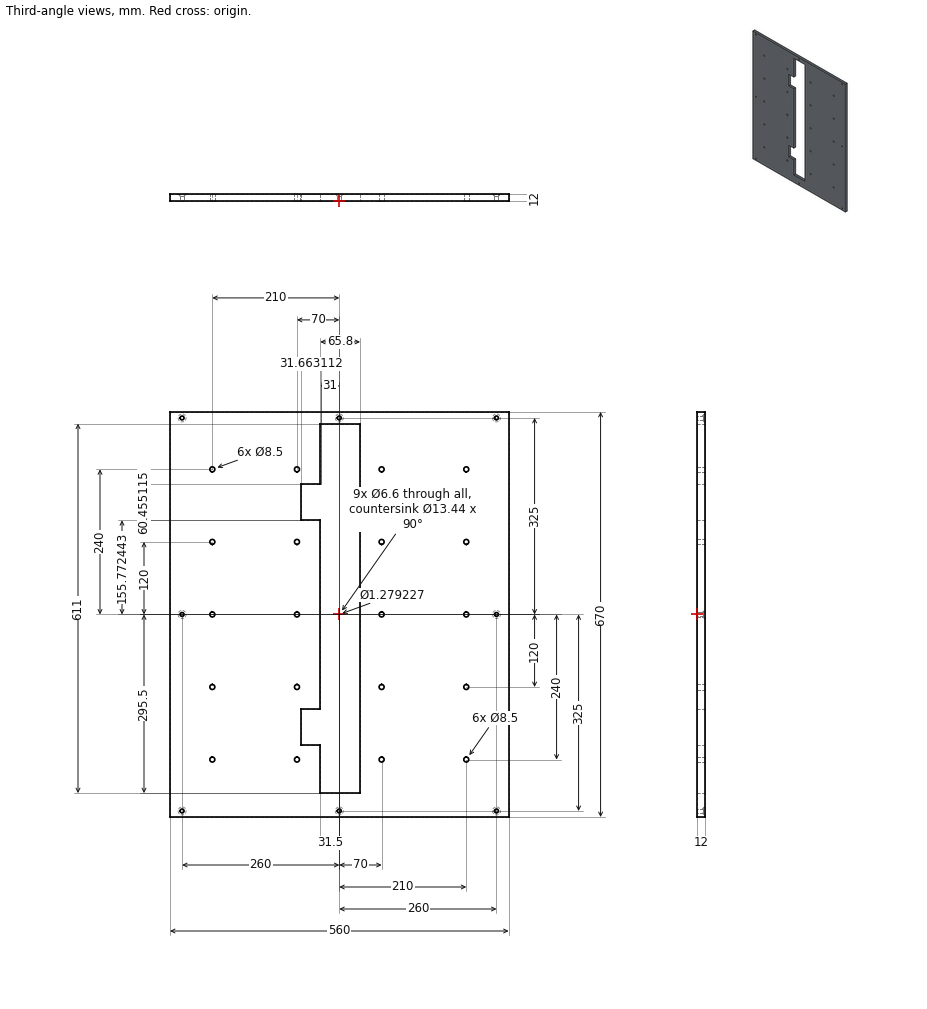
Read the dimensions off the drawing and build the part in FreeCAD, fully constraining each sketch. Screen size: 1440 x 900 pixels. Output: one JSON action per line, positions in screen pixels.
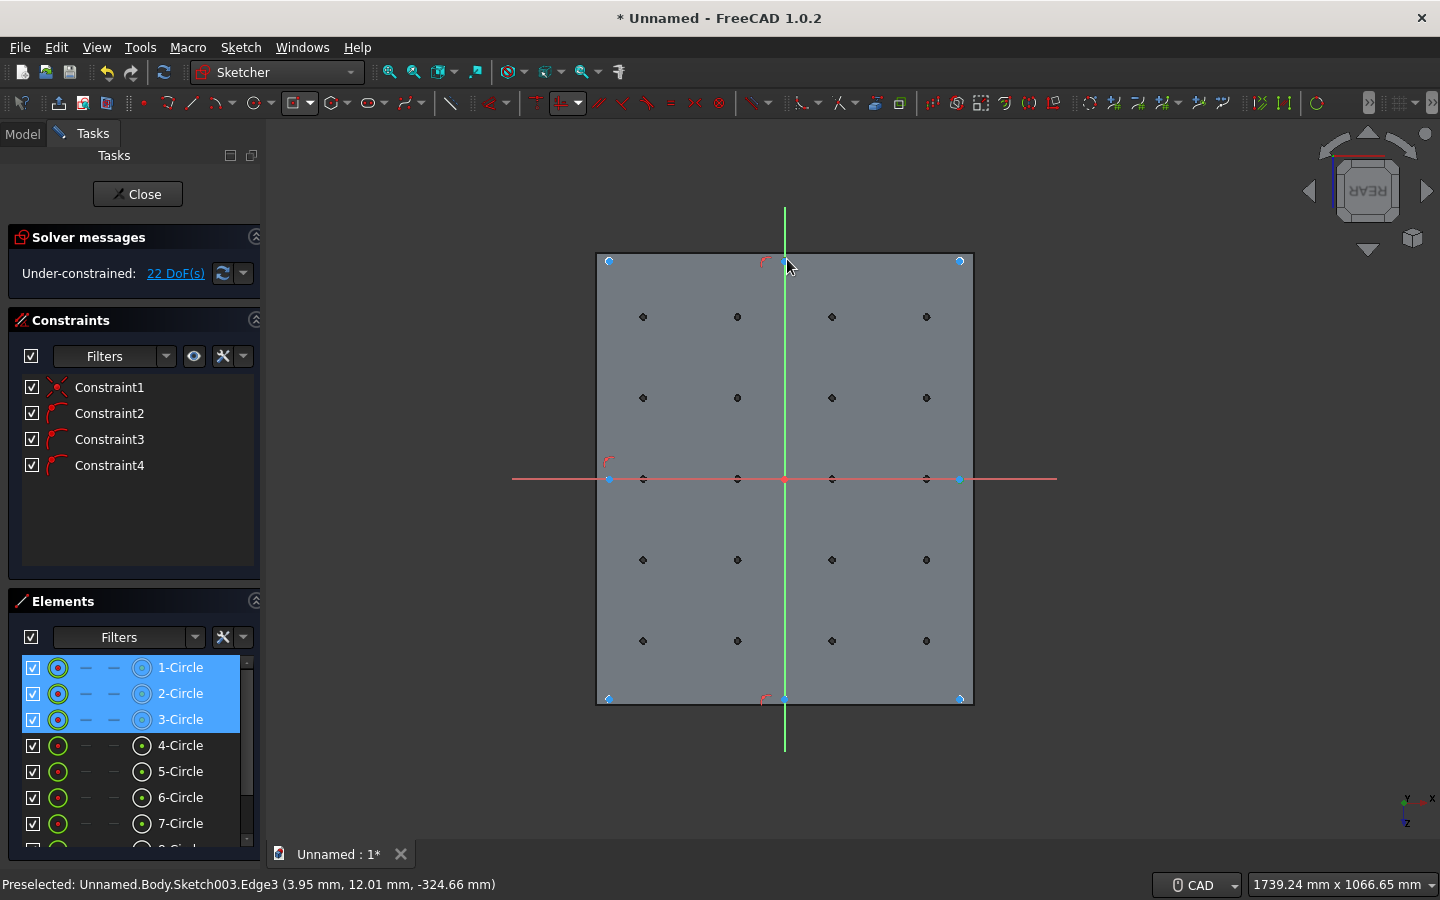
{"action": "scroll", "coordinate": [962, 259], "scroll_direction": "up", "scroll_amount": 8}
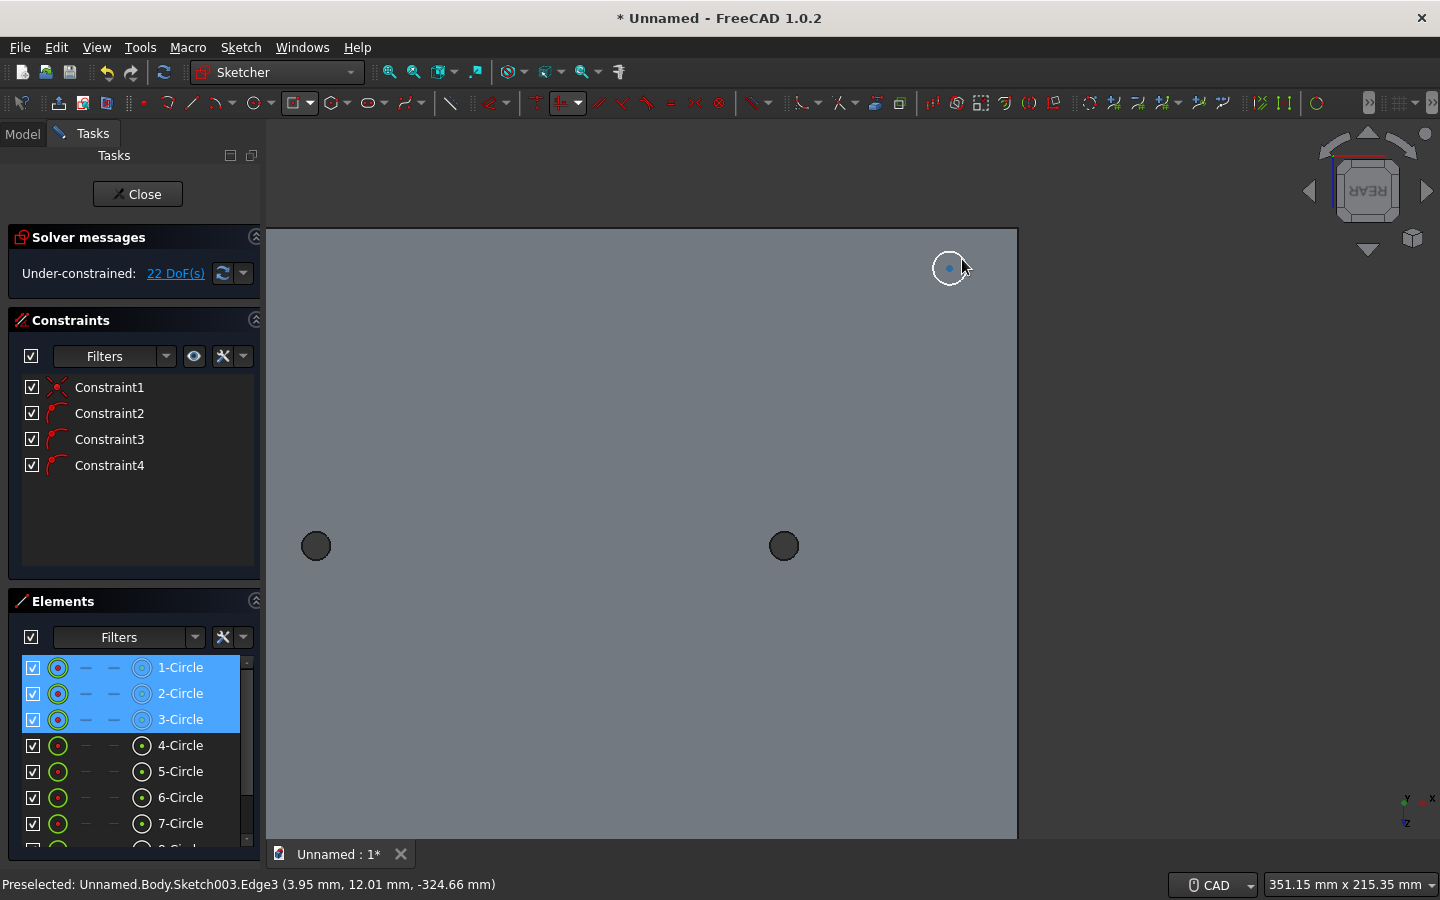
{"action": "left_click", "coordinate": [961, 256]}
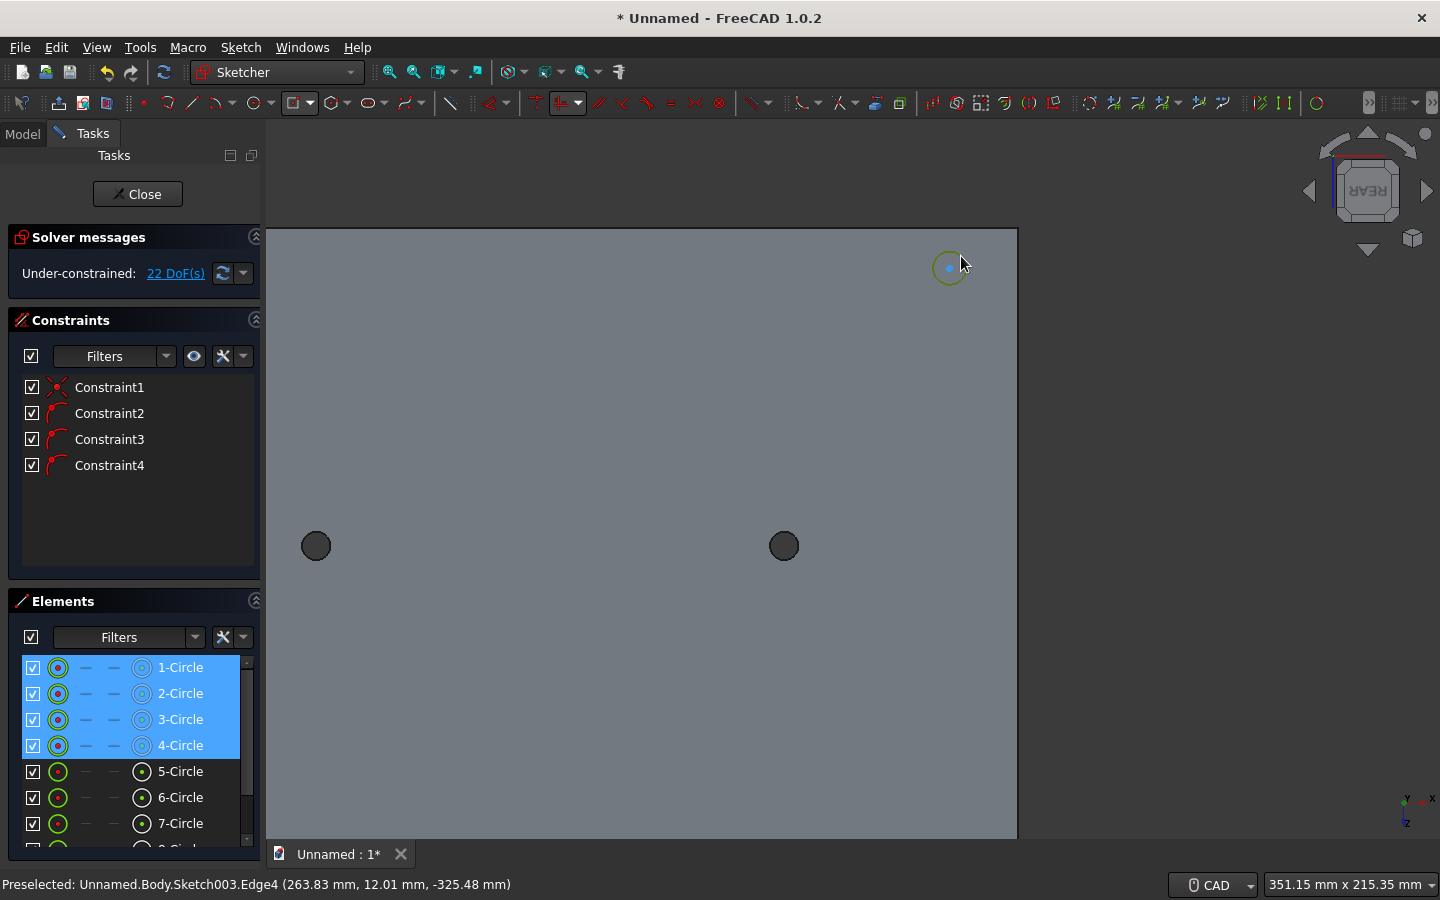
{"action": "scroll", "coordinate": [962, 259], "scroll_direction": "down", "scroll_amount": 8}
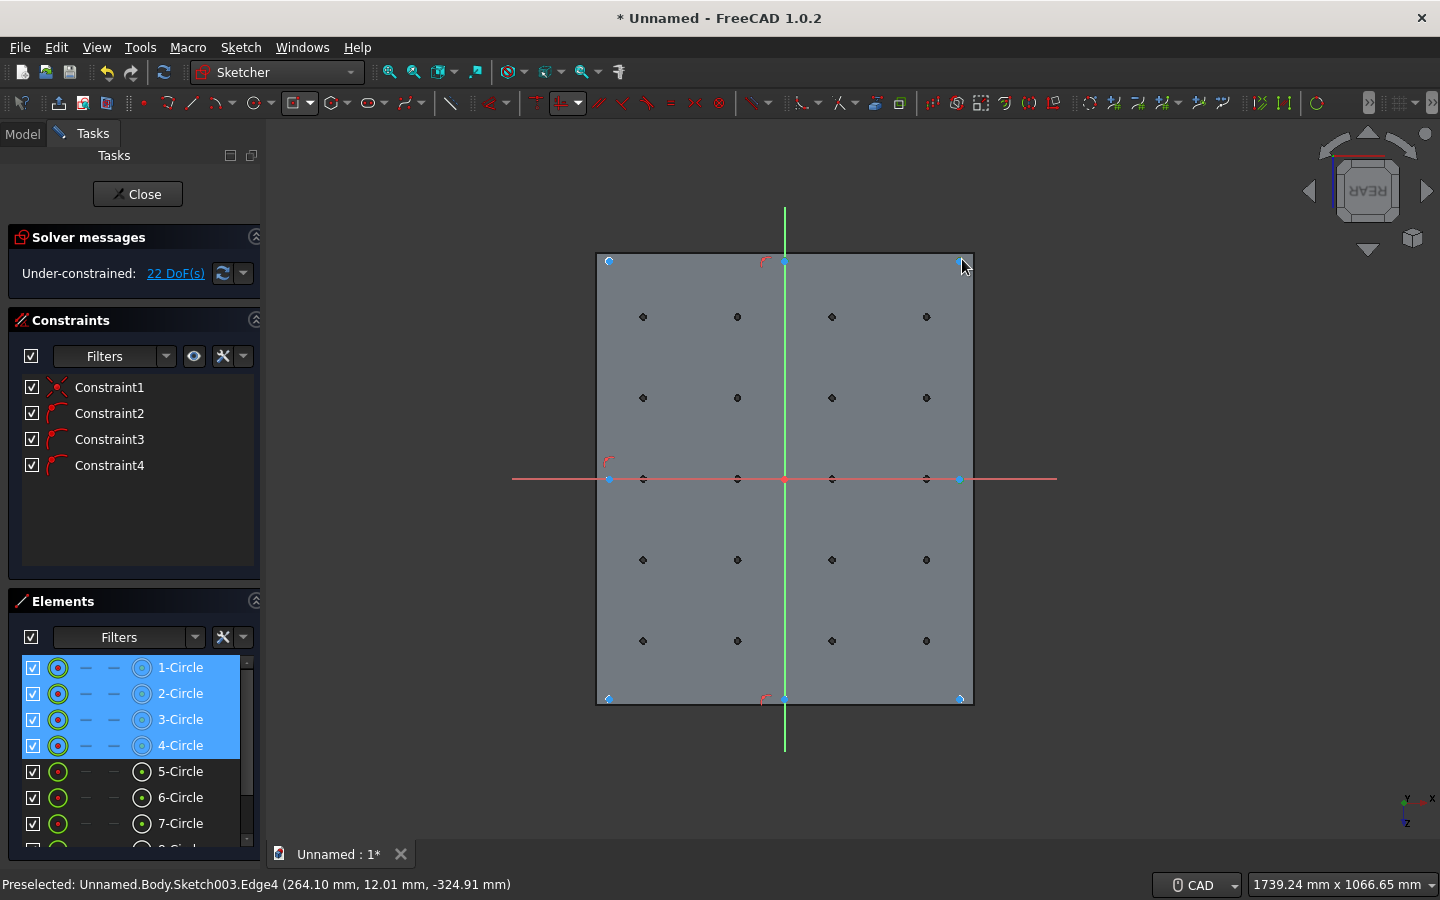
{"action": "scroll", "coordinate": [785, 697], "scroll_direction": "up", "scroll_amount": 9}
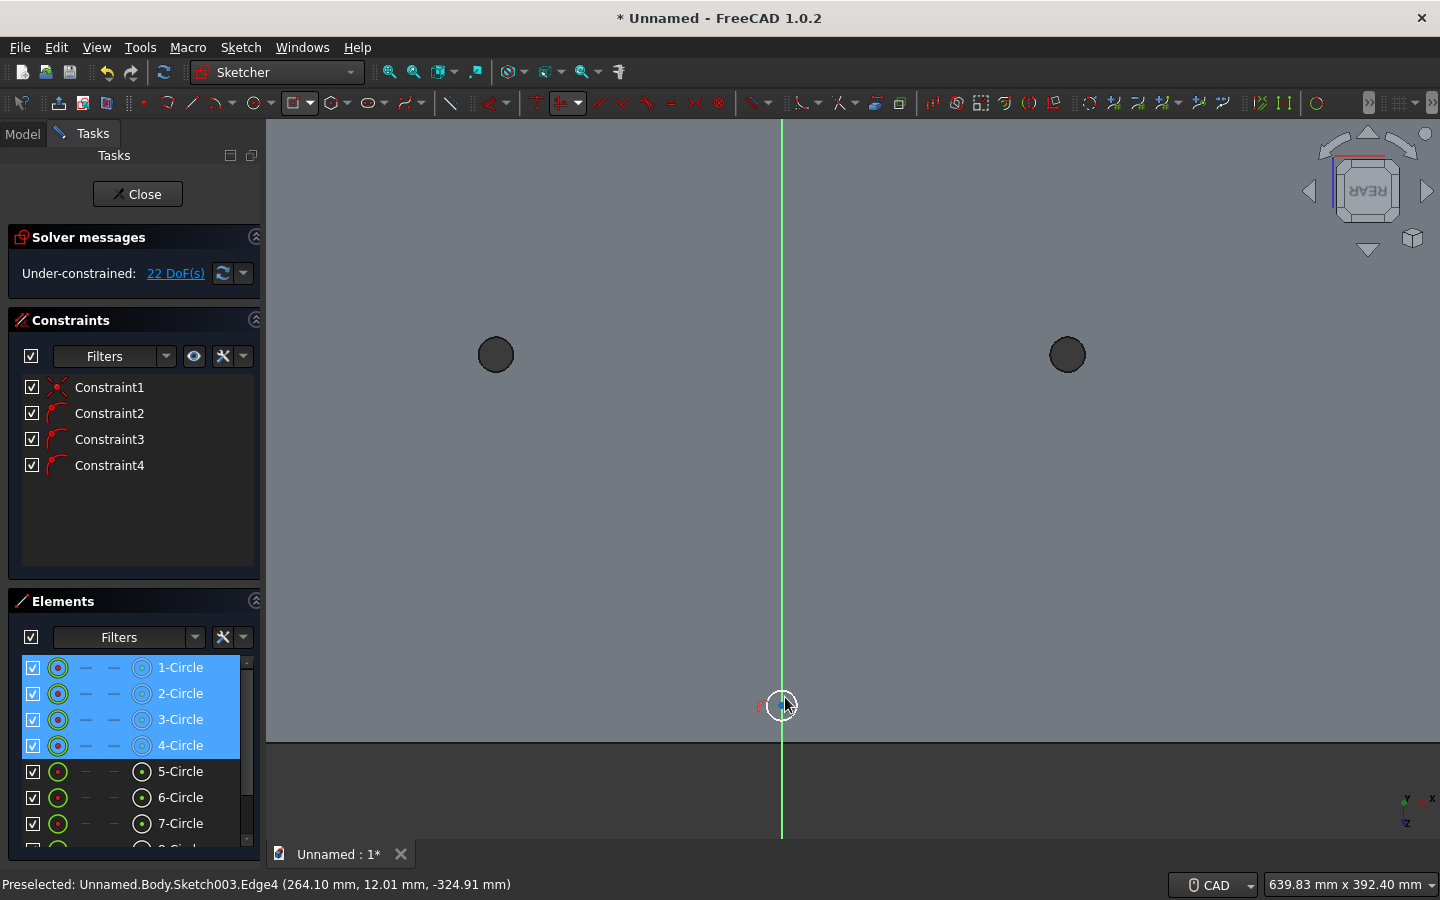
{"action": "left_click", "coordinate": [782, 691]}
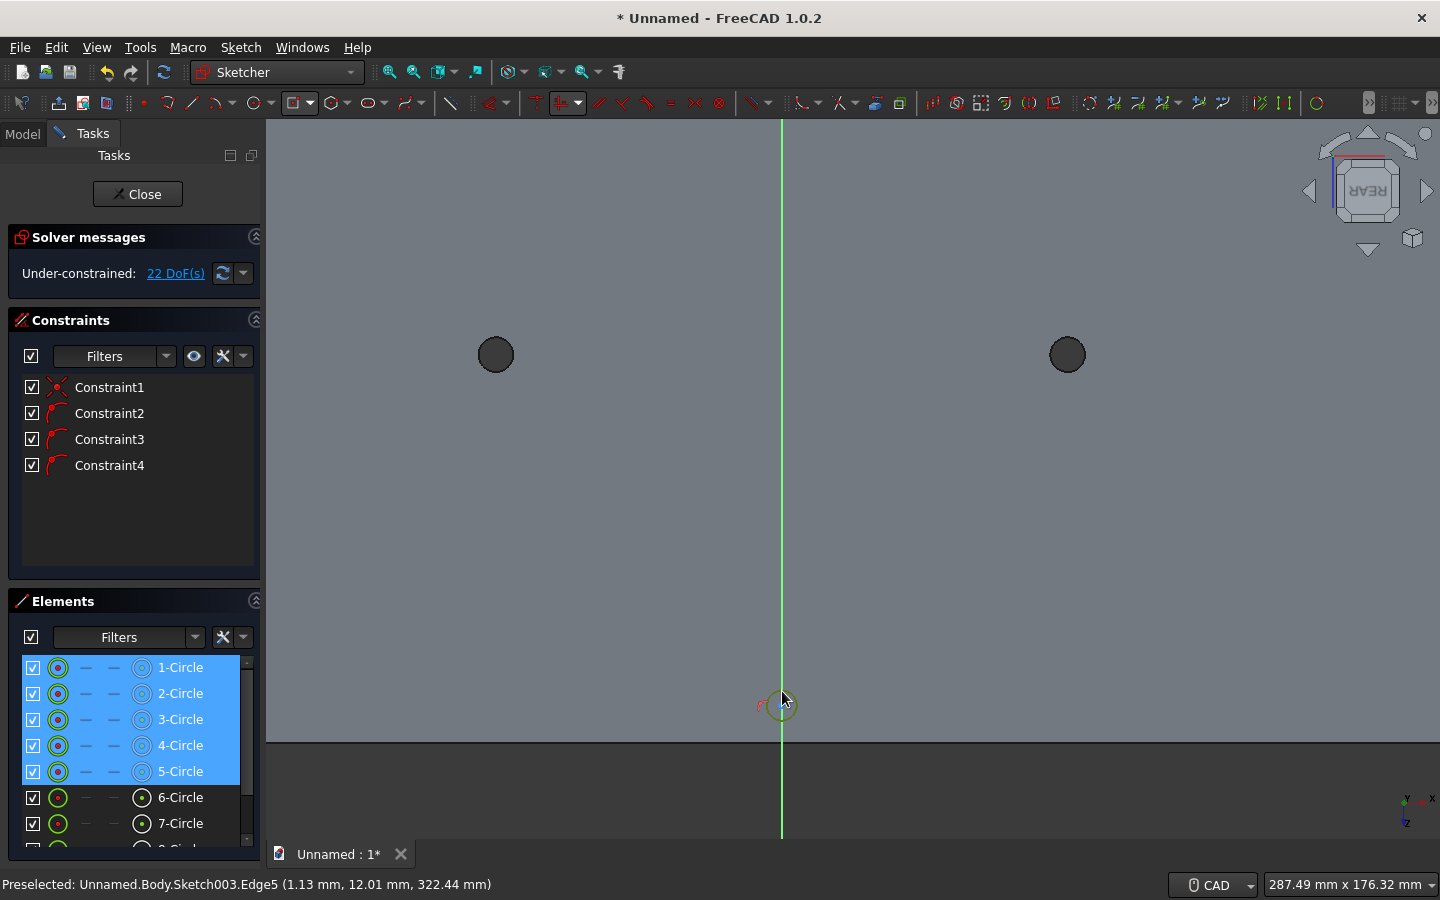
{"action": "scroll", "coordinate": [785, 698], "scroll_direction": "down", "scroll_amount": 9}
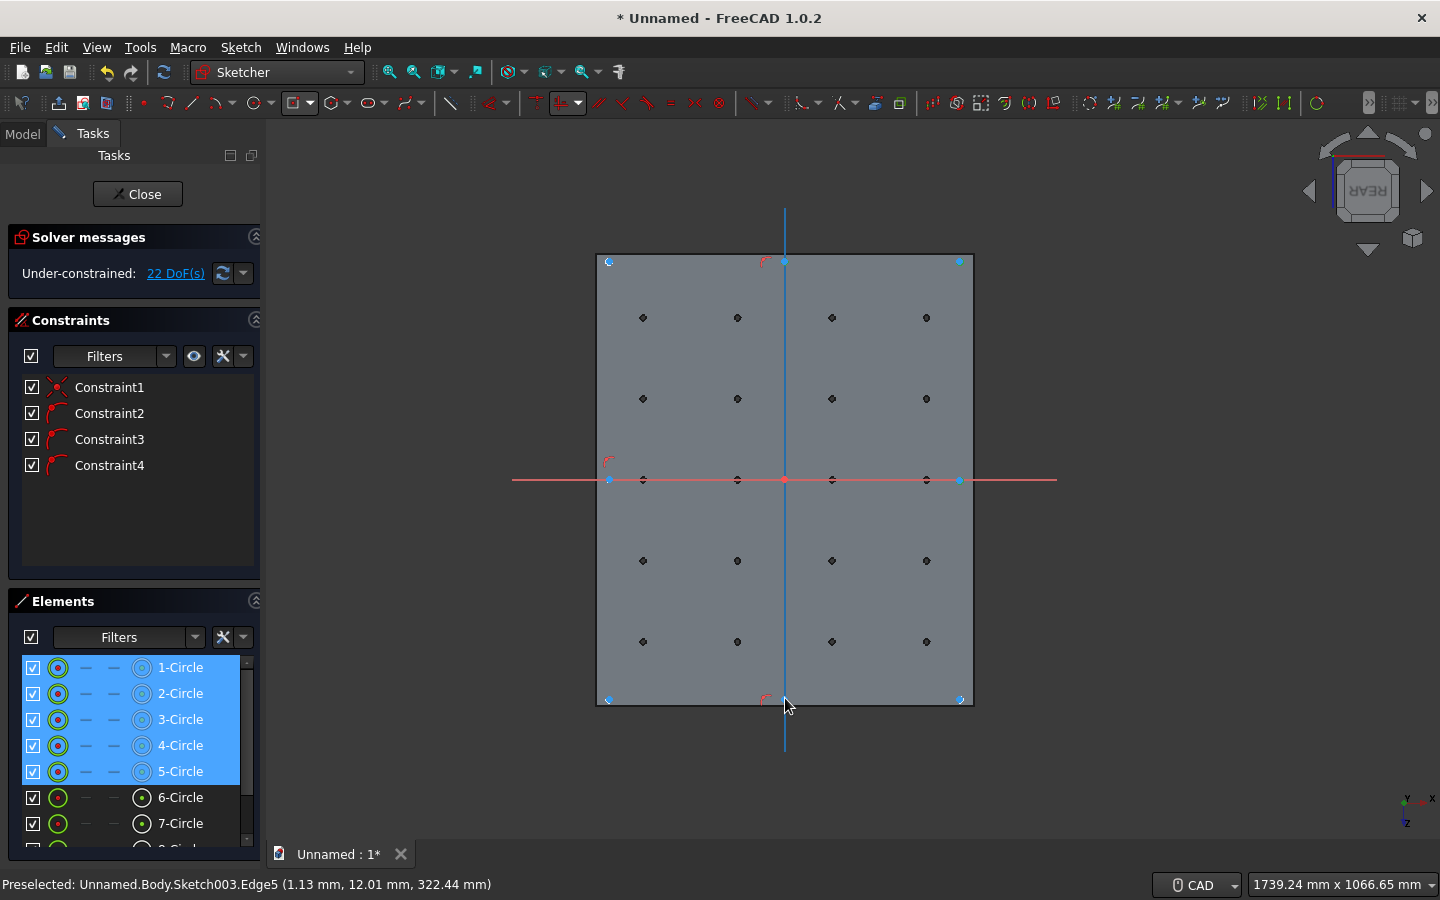
{"action": "scroll", "coordinate": [611, 478], "scroll_direction": "up", "scroll_amount": 11}